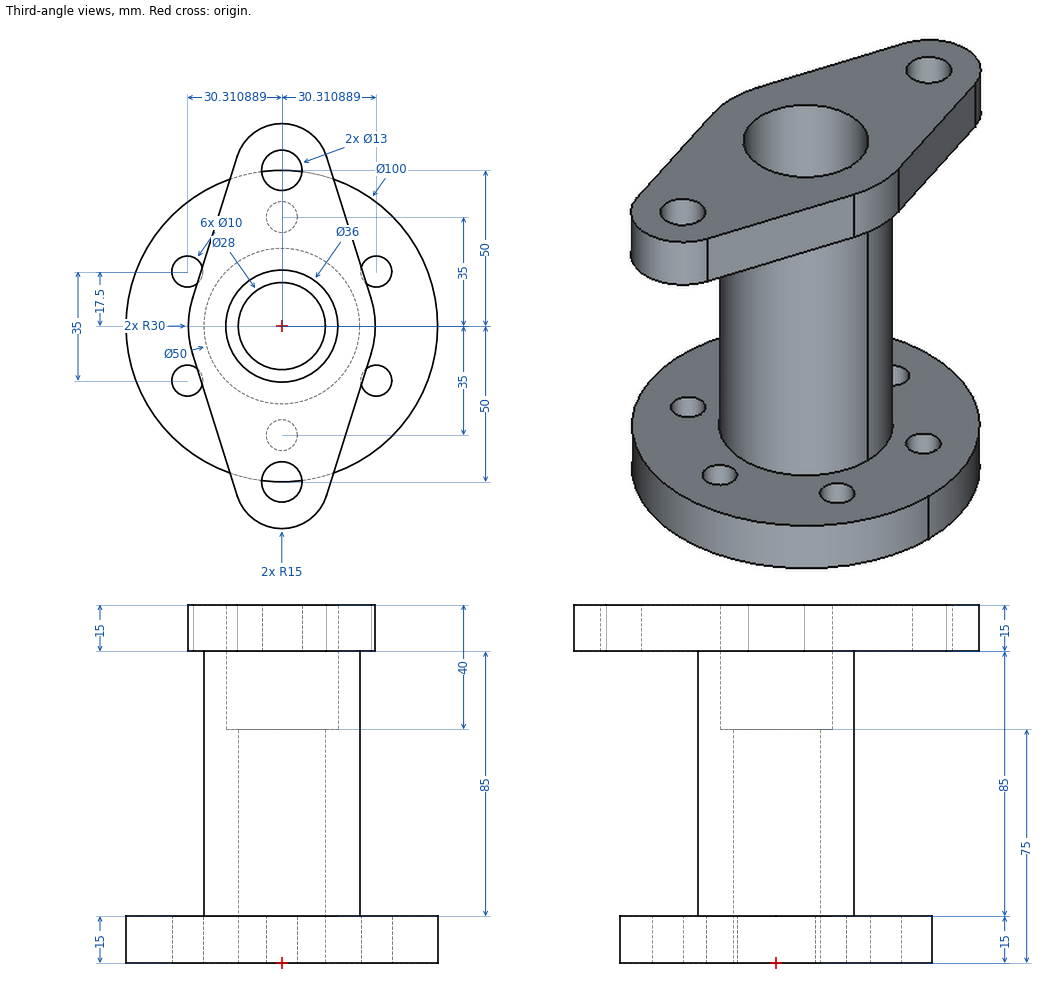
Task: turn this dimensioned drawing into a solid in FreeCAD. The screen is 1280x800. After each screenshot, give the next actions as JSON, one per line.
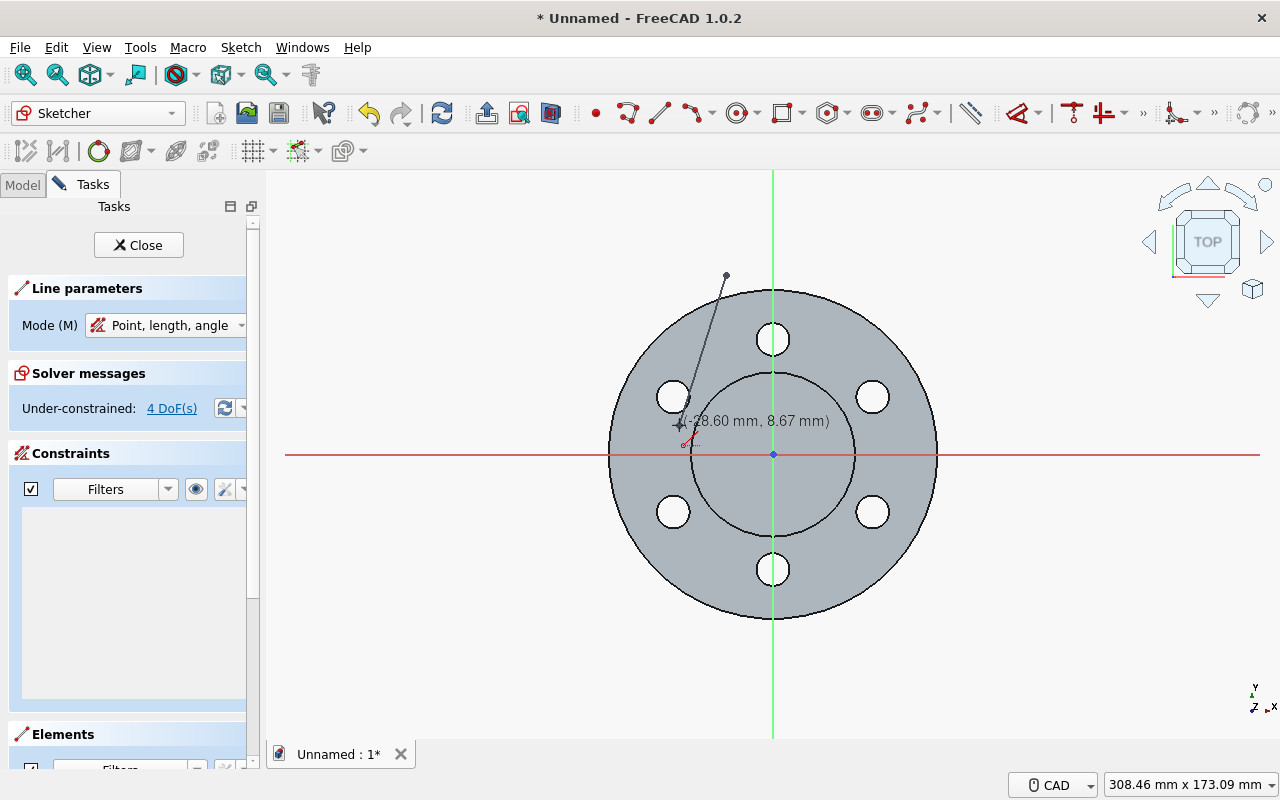
{"action": "left_click", "coordinate": [679, 484]}
{"action": "left_click", "coordinate": [726, 634]}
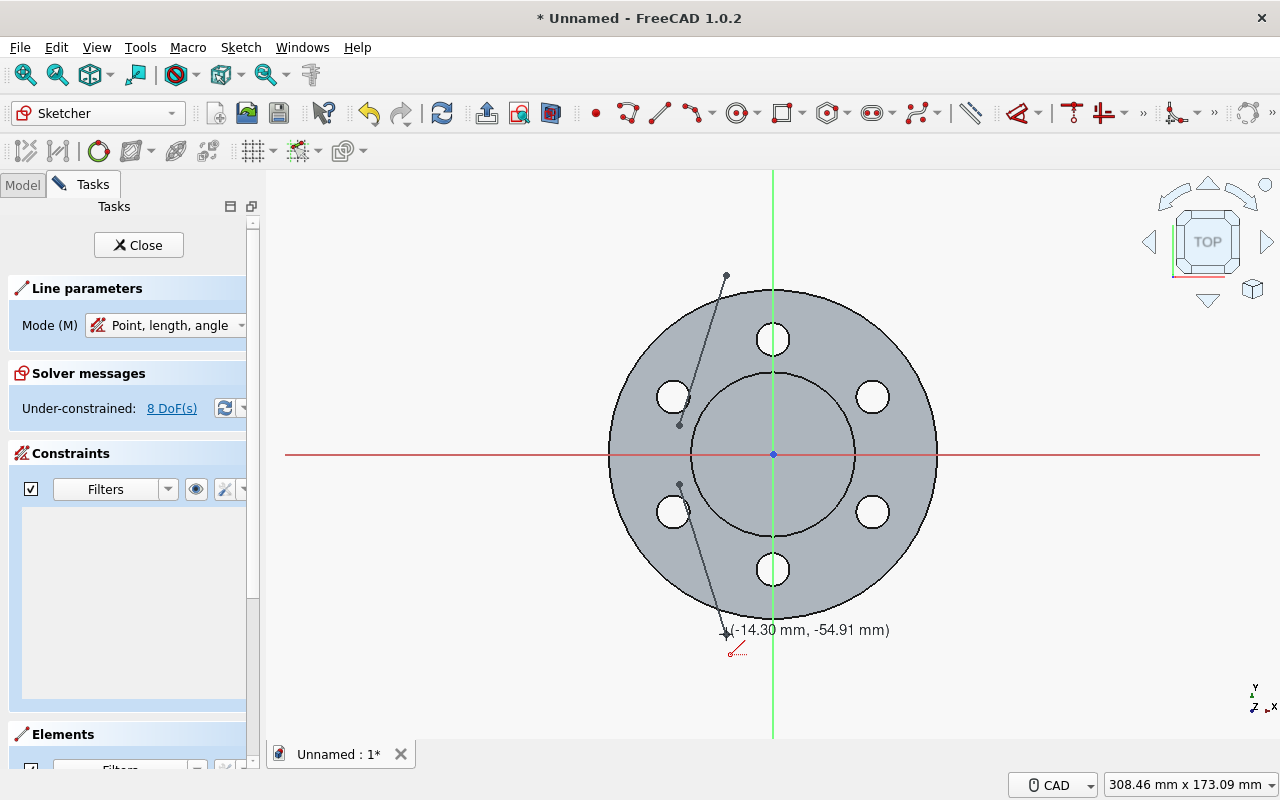
{"action": "left_click", "coordinate": [820, 634]}
{"action": "left_click", "coordinate": [867, 484]}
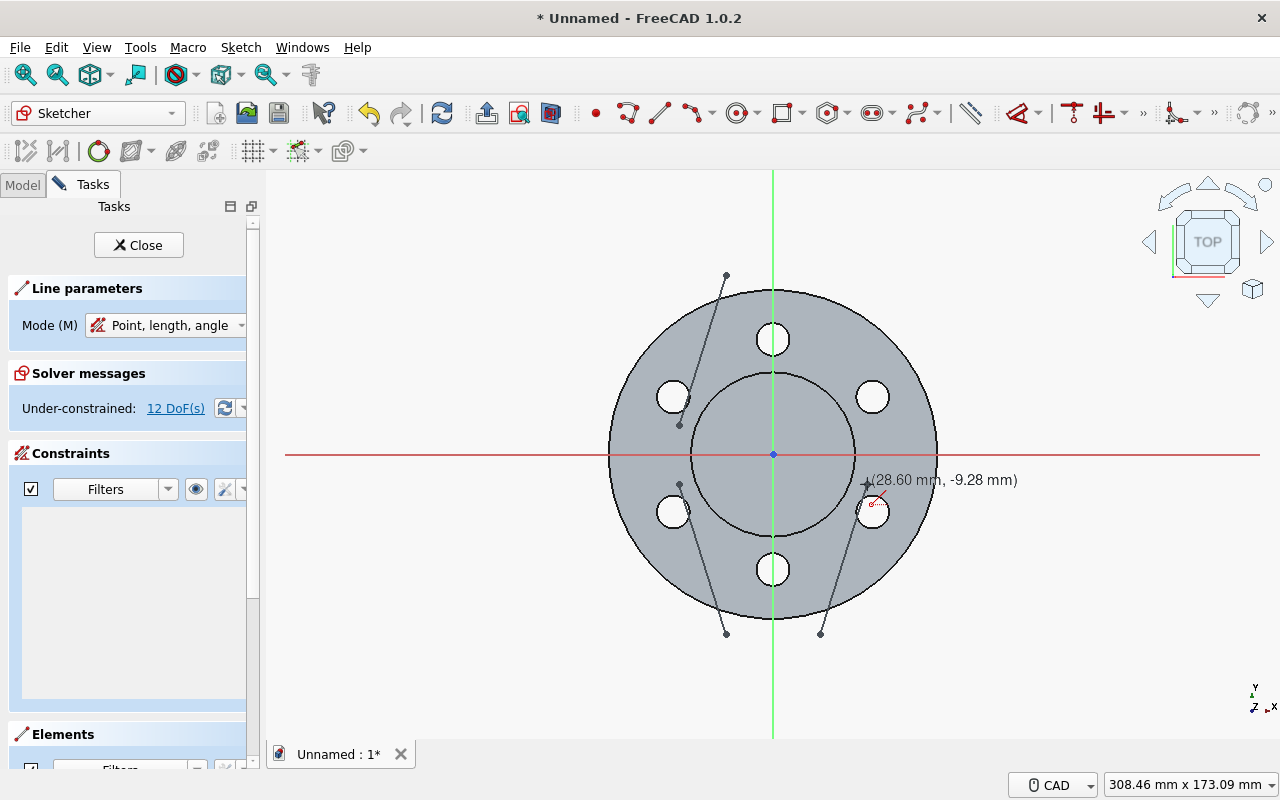
{"action": "left_click", "coordinate": [867, 425]}
{"action": "left_click", "coordinate": [820, 275]}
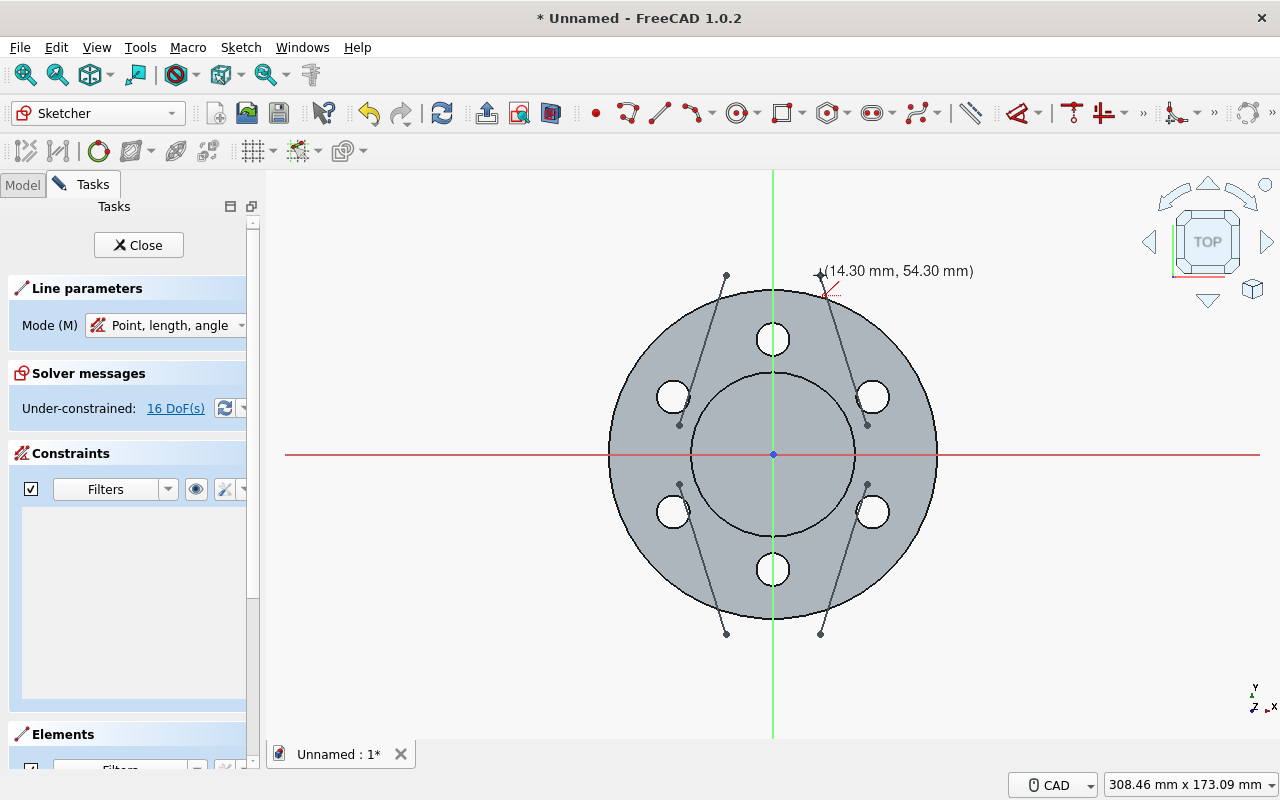
{"action": "key", "text": "g 3 a"}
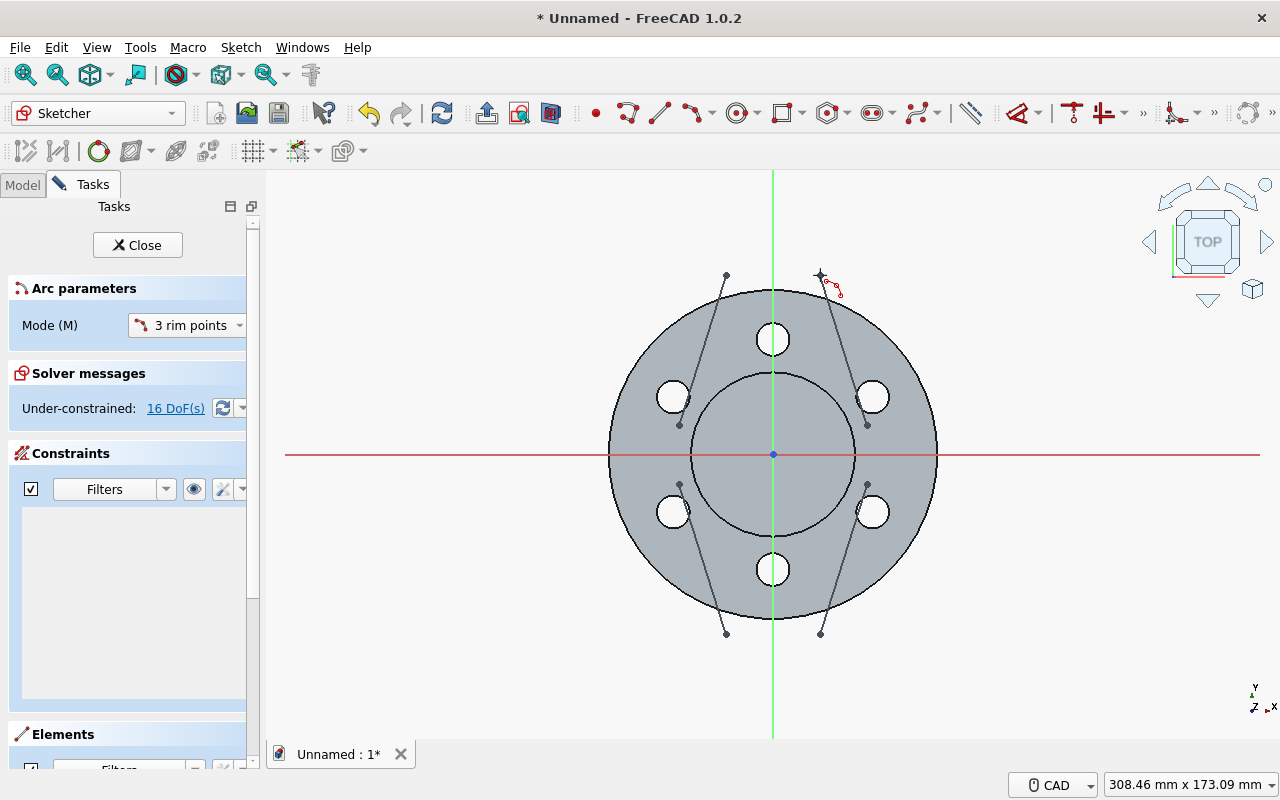
{"action": "left_click", "coordinate": [679, 426]}
{"action": "left_click", "coordinate": [679, 485]}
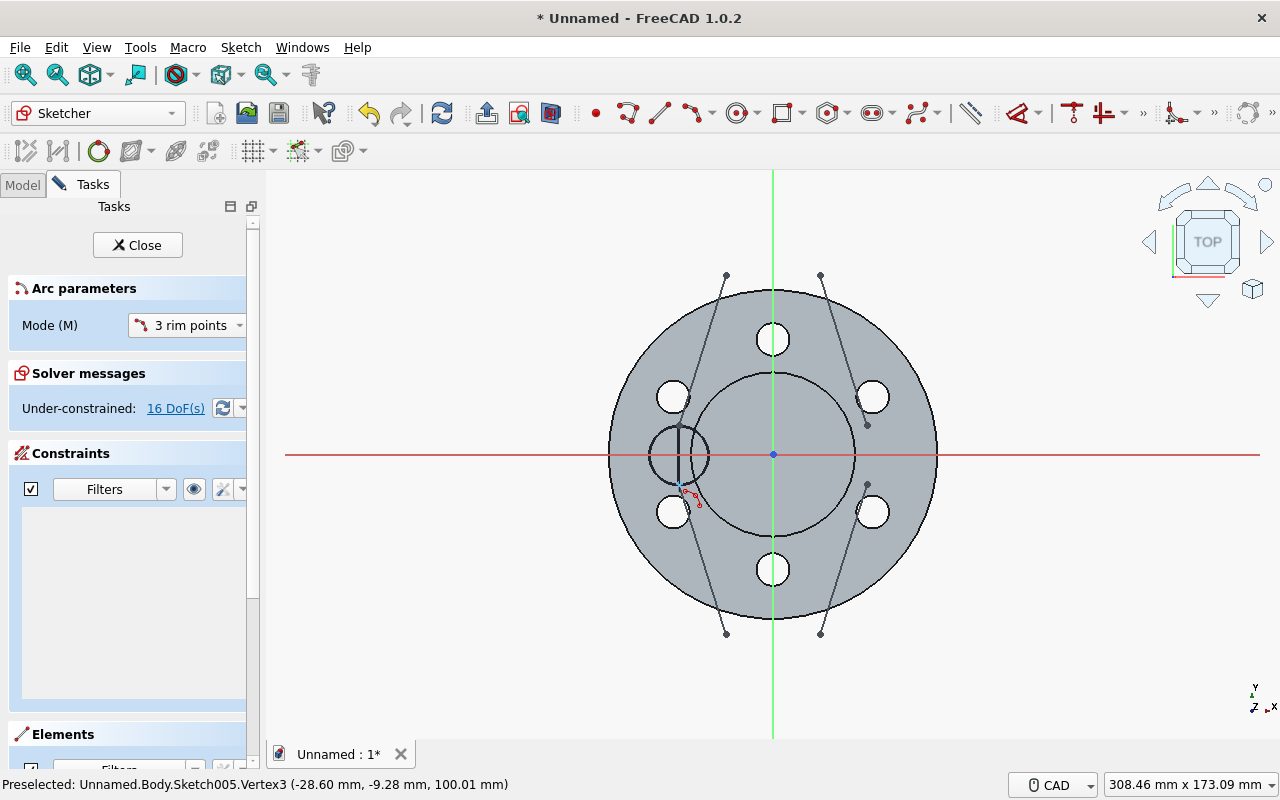
{"action": "scroll", "coordinate": [675, 448], "scroll_direction": "up", "scroll_amount": 7}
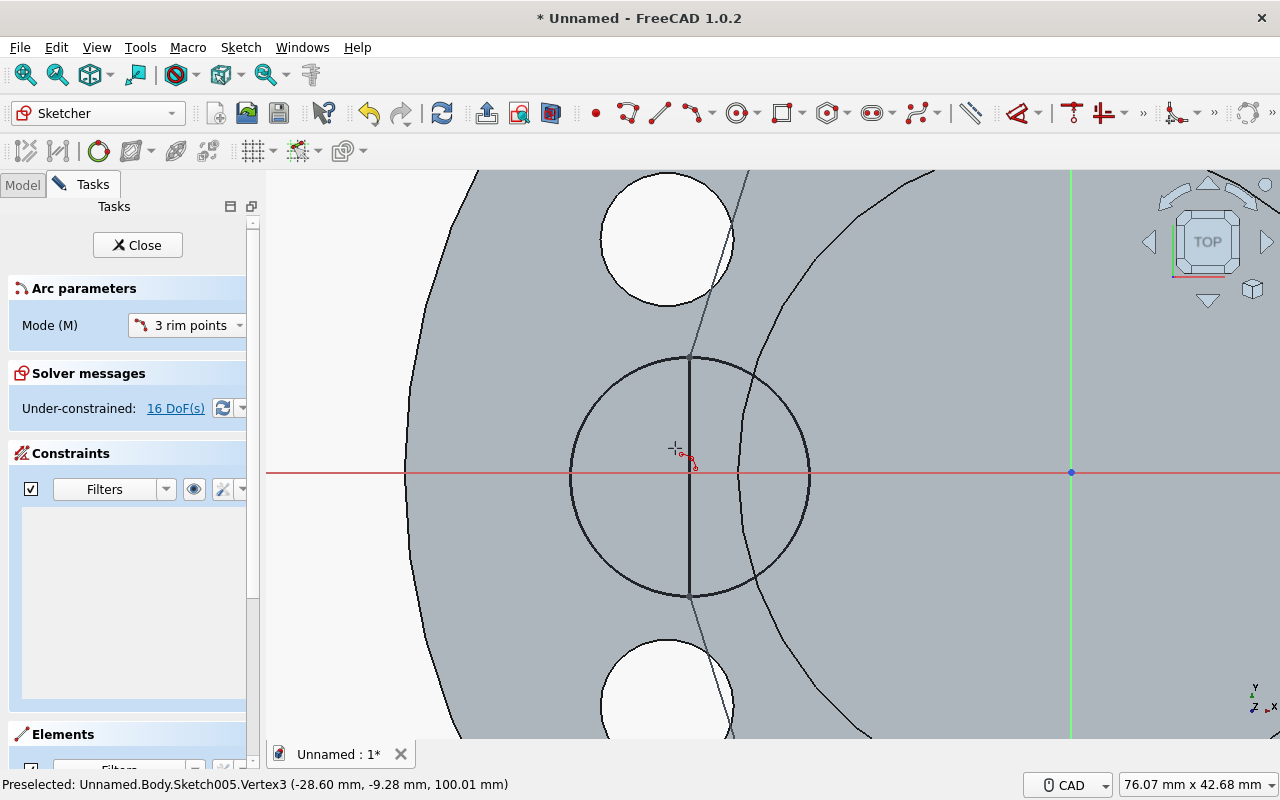
{"action": "left_click", "coordinate": [672, 449]}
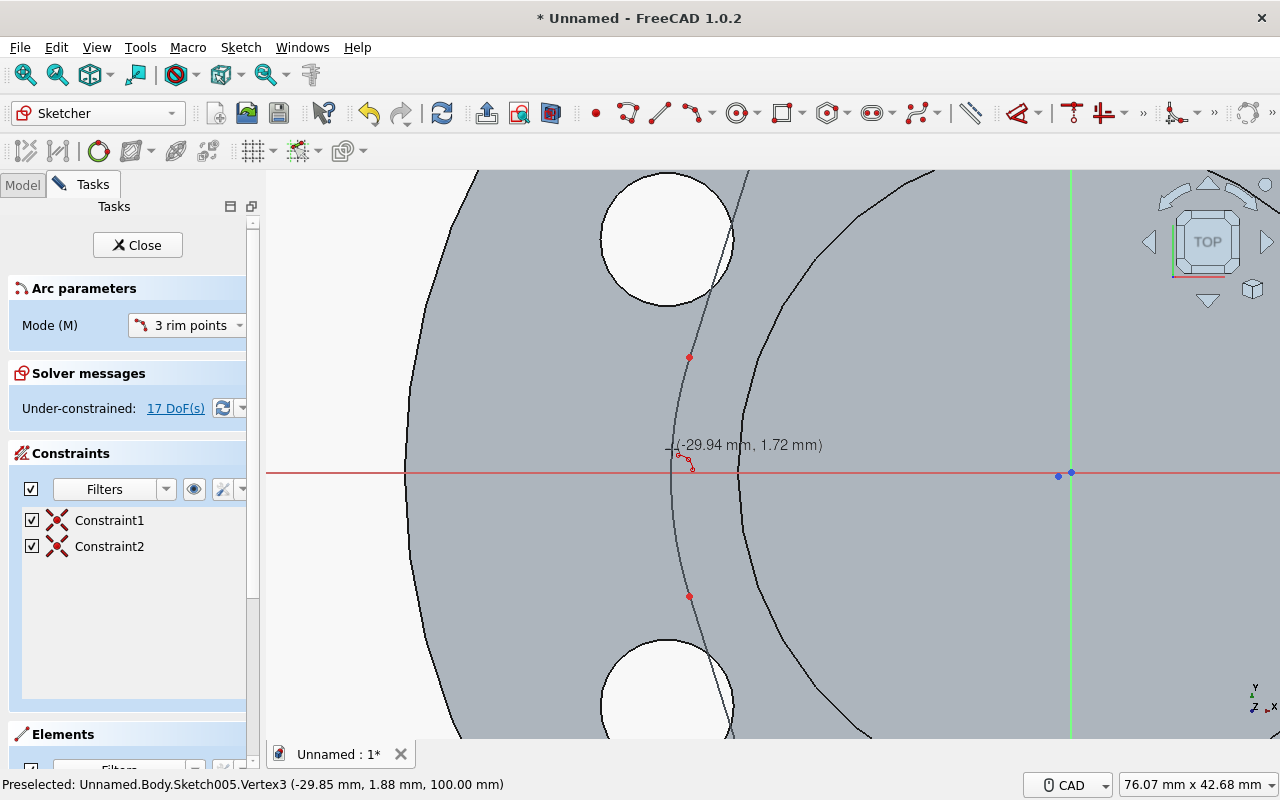
{"action": "scroll", "coordinate": [612, 450], "scroll_direction": "down", "scroll_amount": 8}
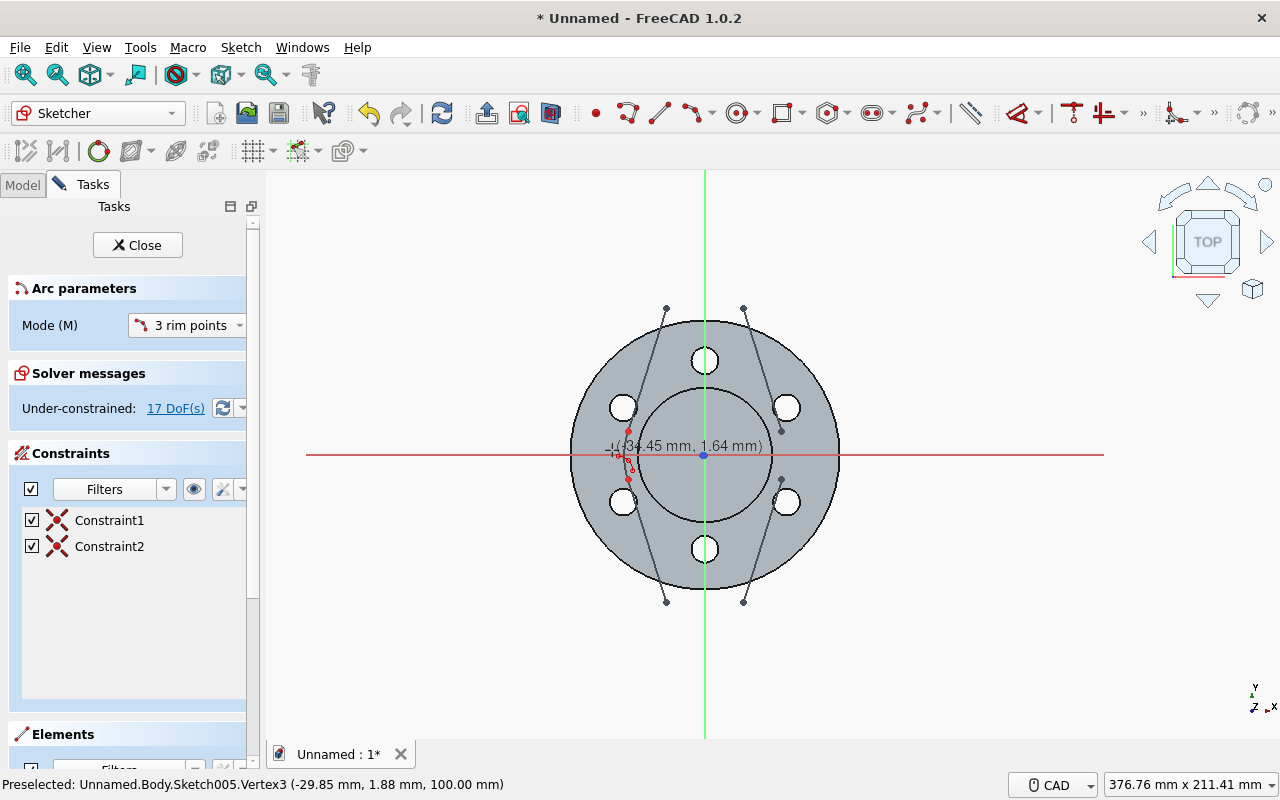
{"action": "left_click", "coordinate": [666, 603]}
{"action": "left_click", "coordinate": [743, 603]}
{"action": "left_click", "coordinate": [685, 625]}